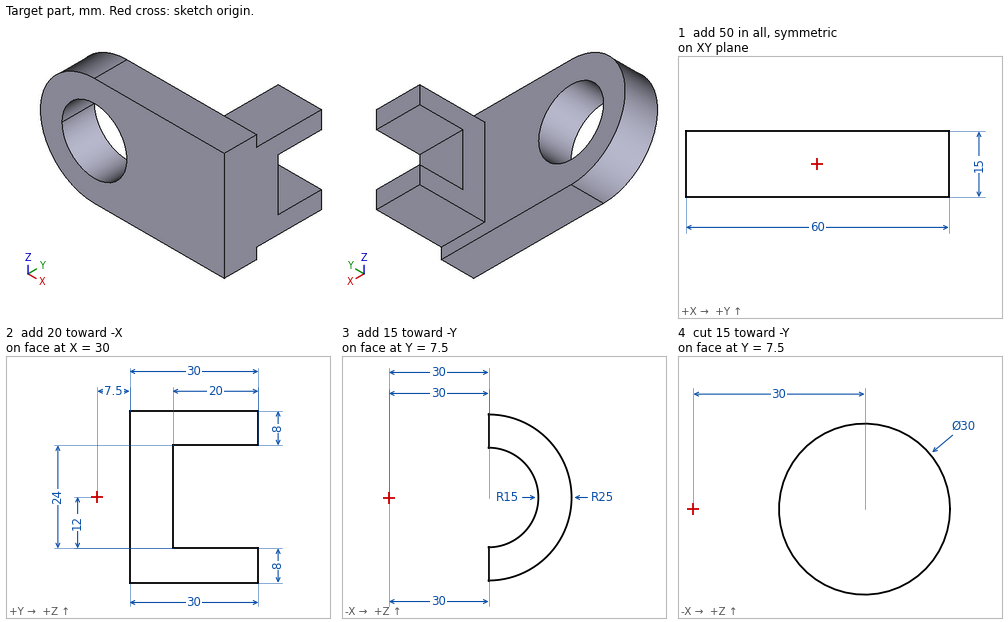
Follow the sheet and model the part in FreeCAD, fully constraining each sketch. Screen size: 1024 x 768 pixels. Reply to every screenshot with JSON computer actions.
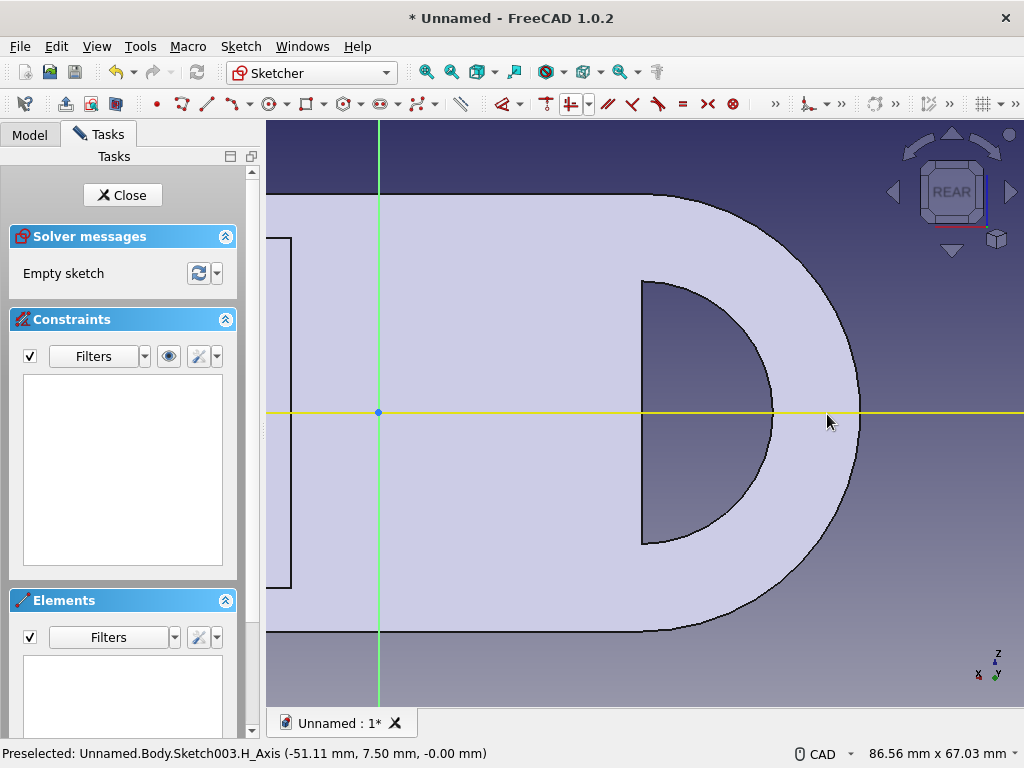
{"action": "key", "text": "g c"}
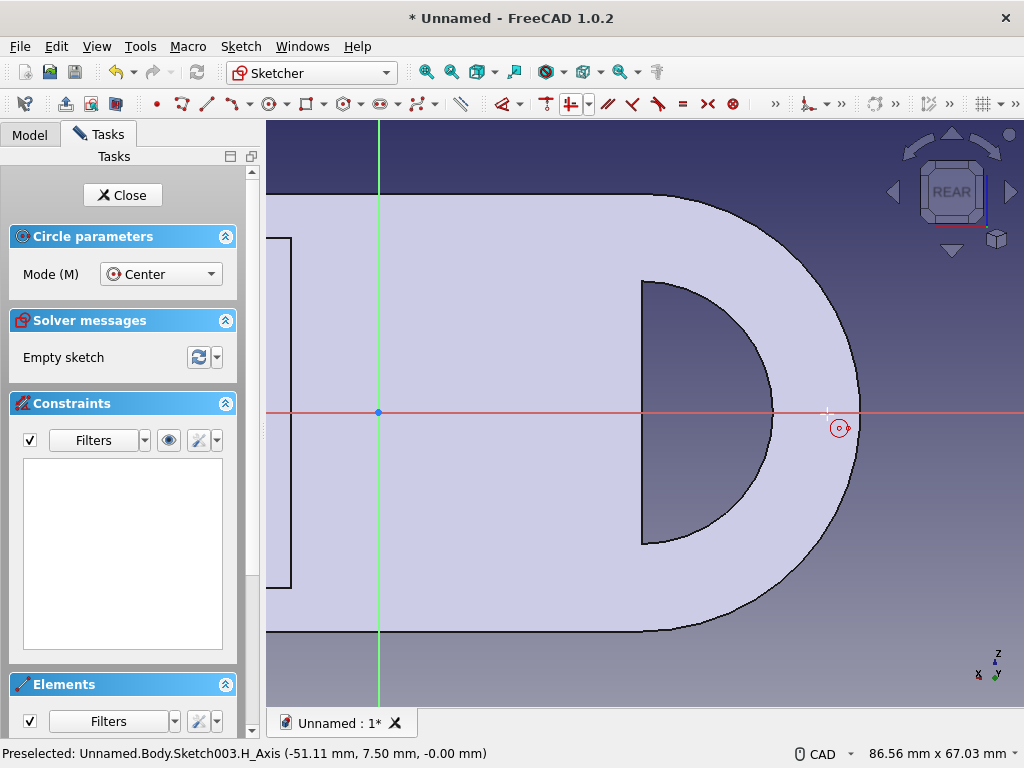
{"action": "left_click", "coordinate": [642, 413]}
{"action": "mouse_move", "coordinate": [734, 320]}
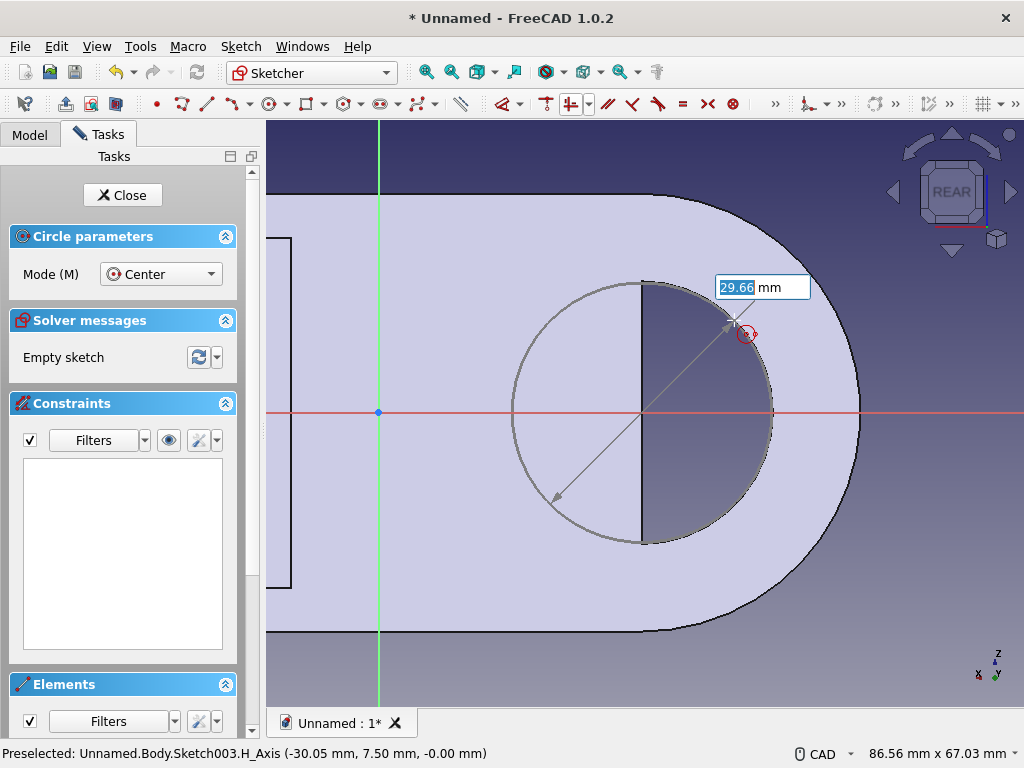
{"action": "type", "text": "30"}
{"action": "key", "text": "Return"}
{"action": "key", "text": "Escape"}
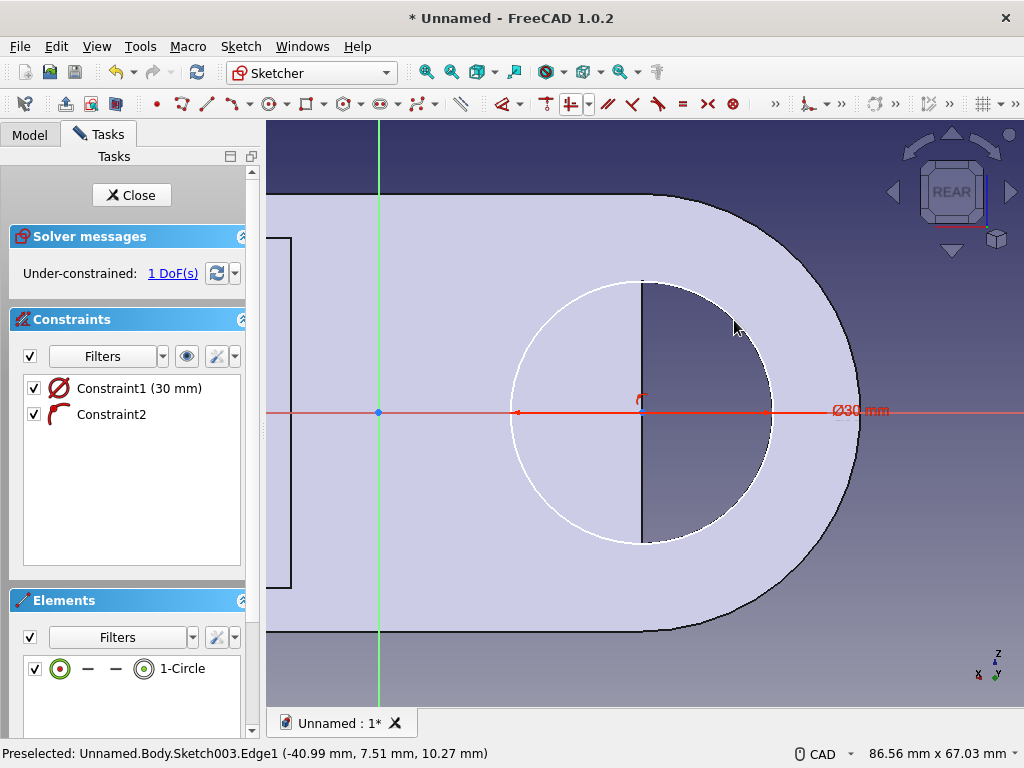
{"action": "key", "text": "d"}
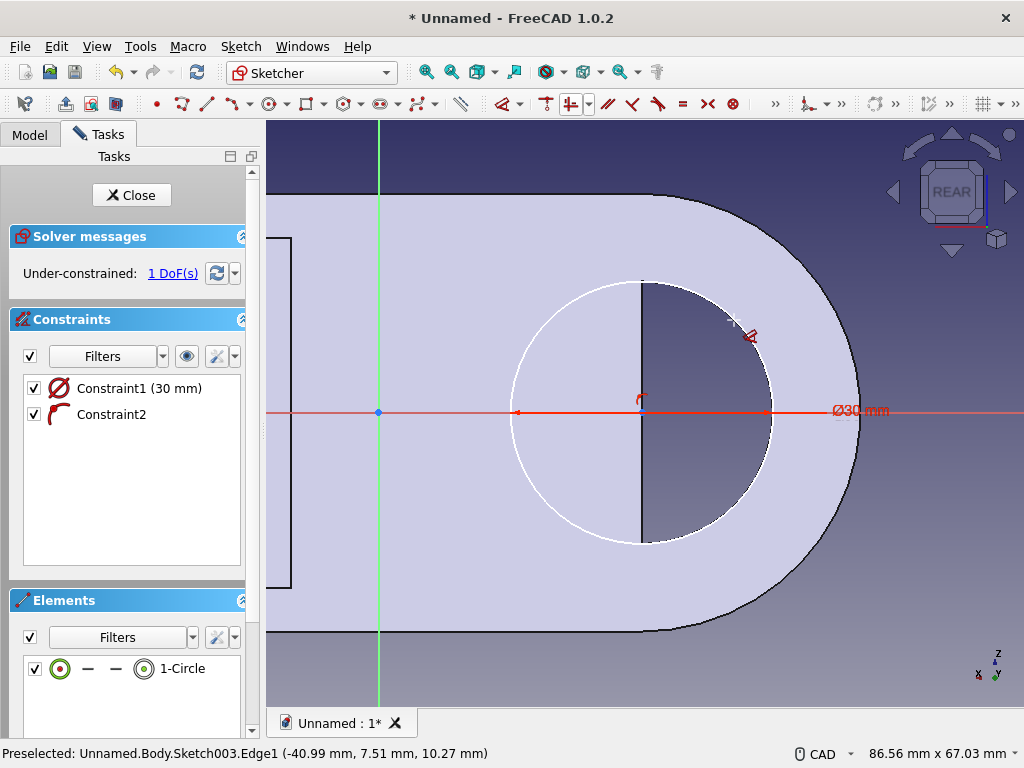
{"action": "left_click", "coordinate": [642, 413]}
{"action": "left_click", "coordinate": [450, 447]}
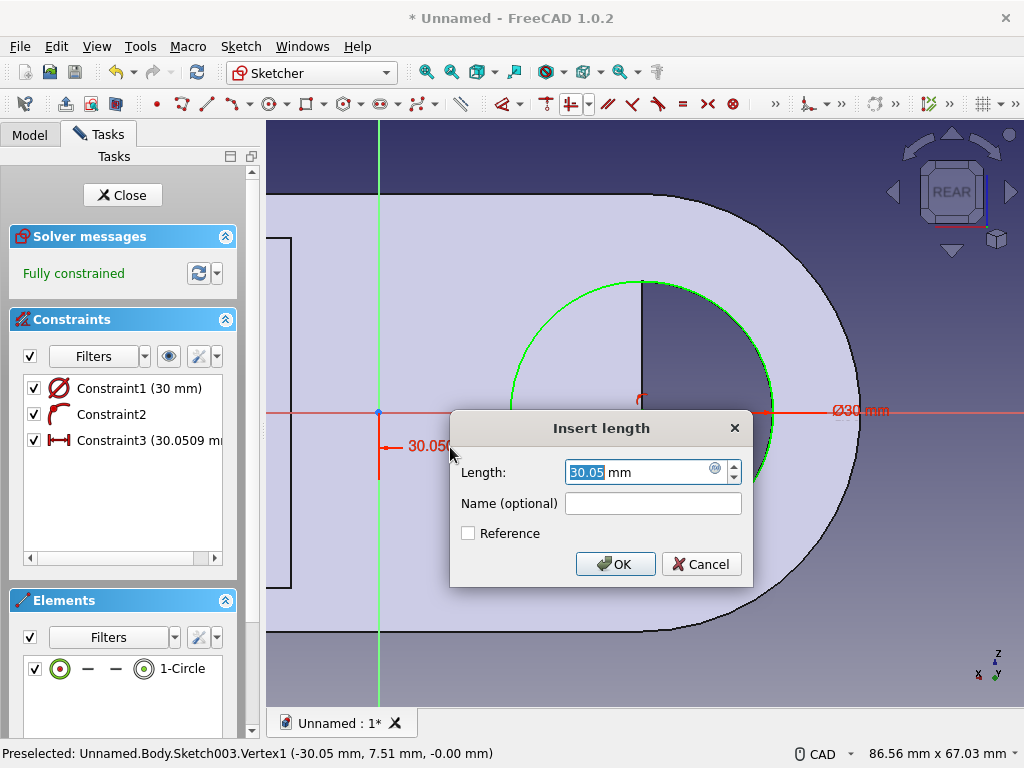
{"action": "type", "text": "30"}
{"action": "key", "text": "Return"}
{"action": "key", "text": "Escape"}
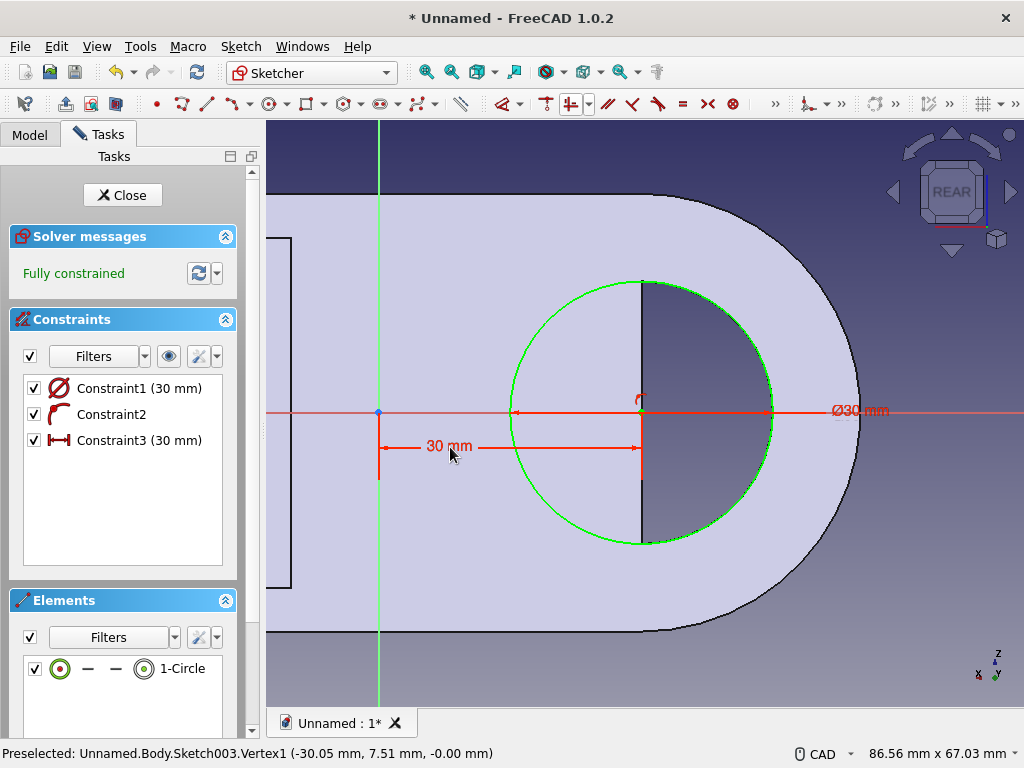
{"action": "left_click", "coordinate": [123, 195]}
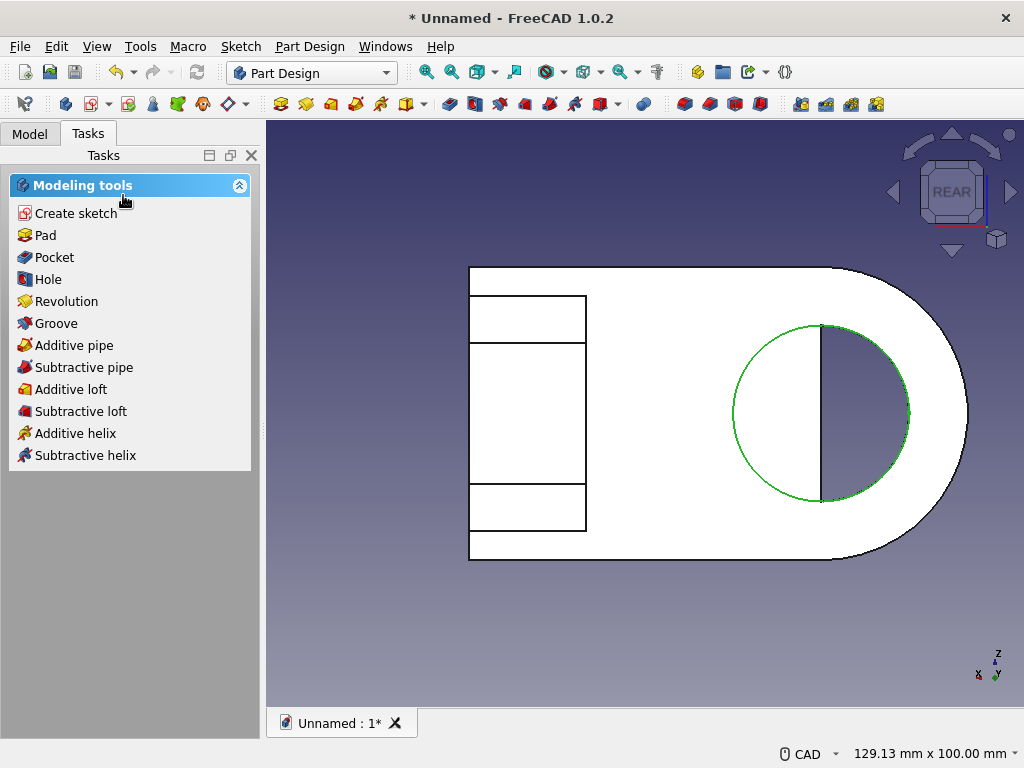
{"action": "left_click", "coordinate": [450, 104]}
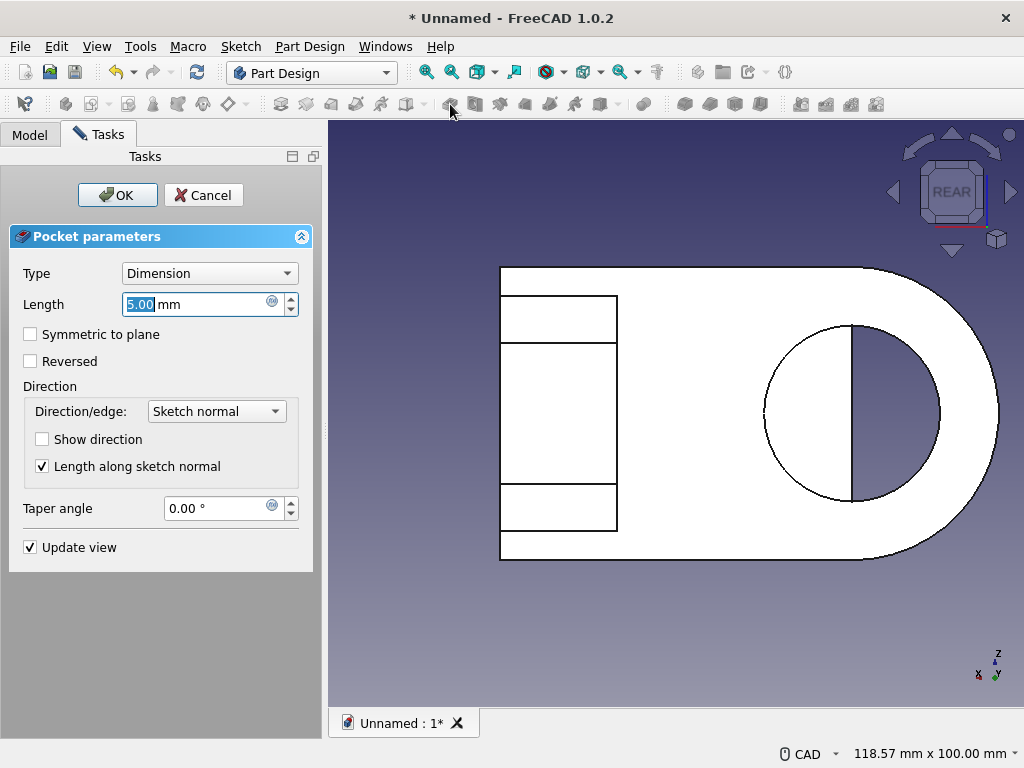
{"action": "type", "text": "15"}
{"action": "key", "text": "Tab"}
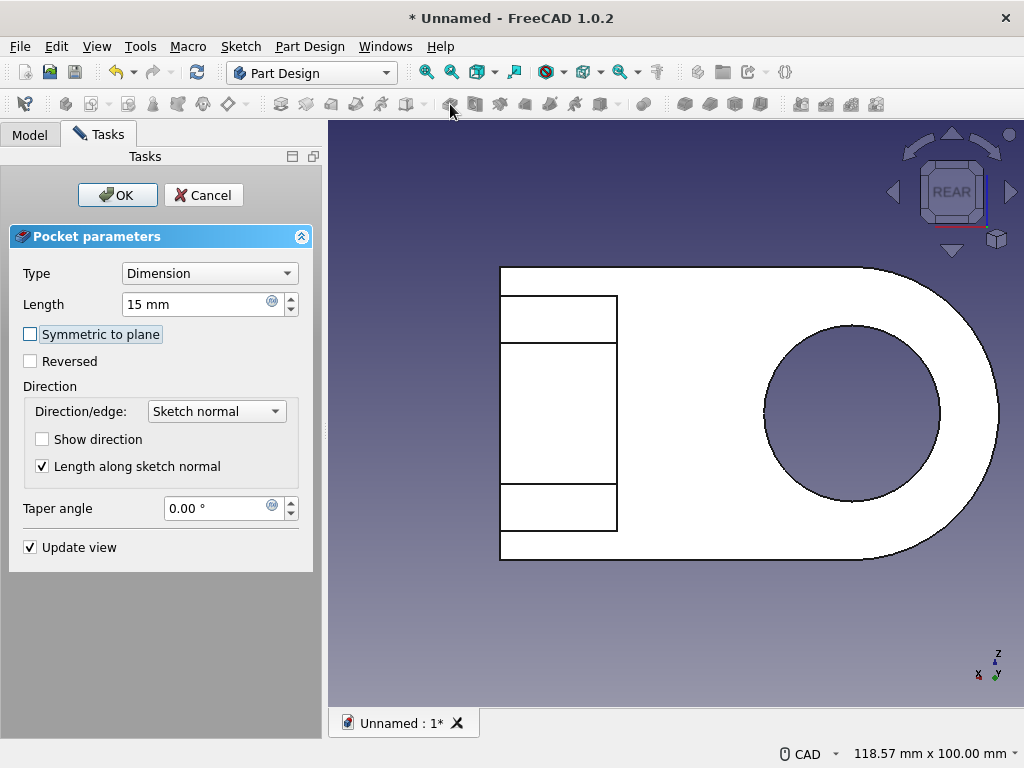
{"action": "left_click", "coordinate": [118, 195]}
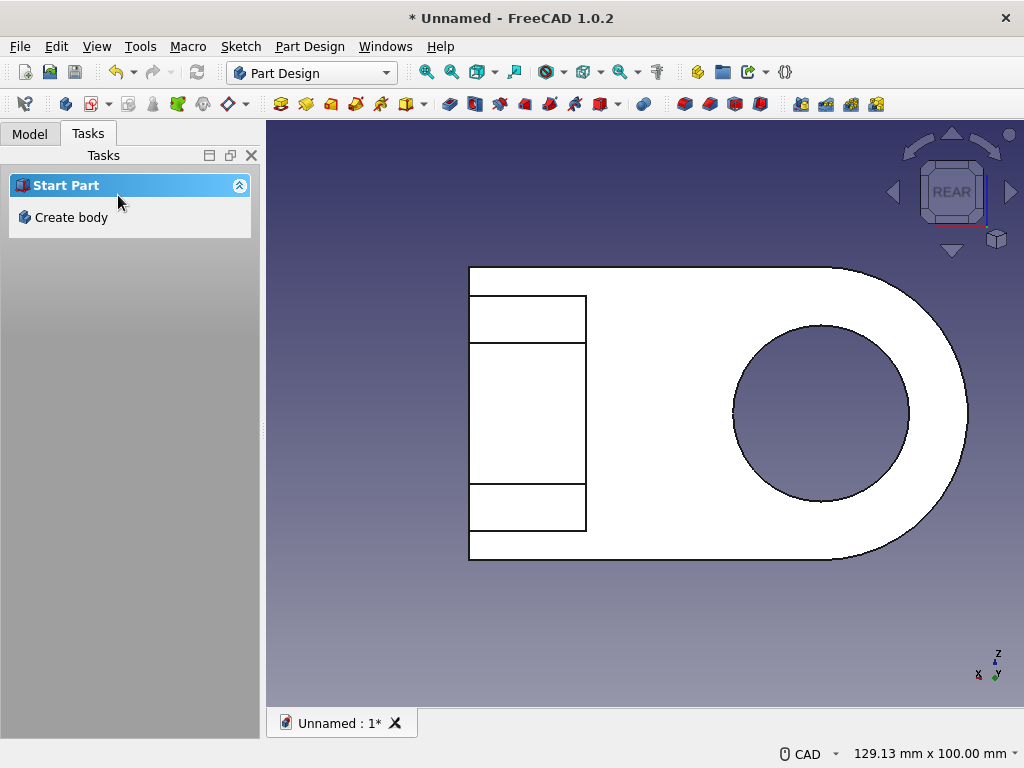
{"action": "key", "text": "0"}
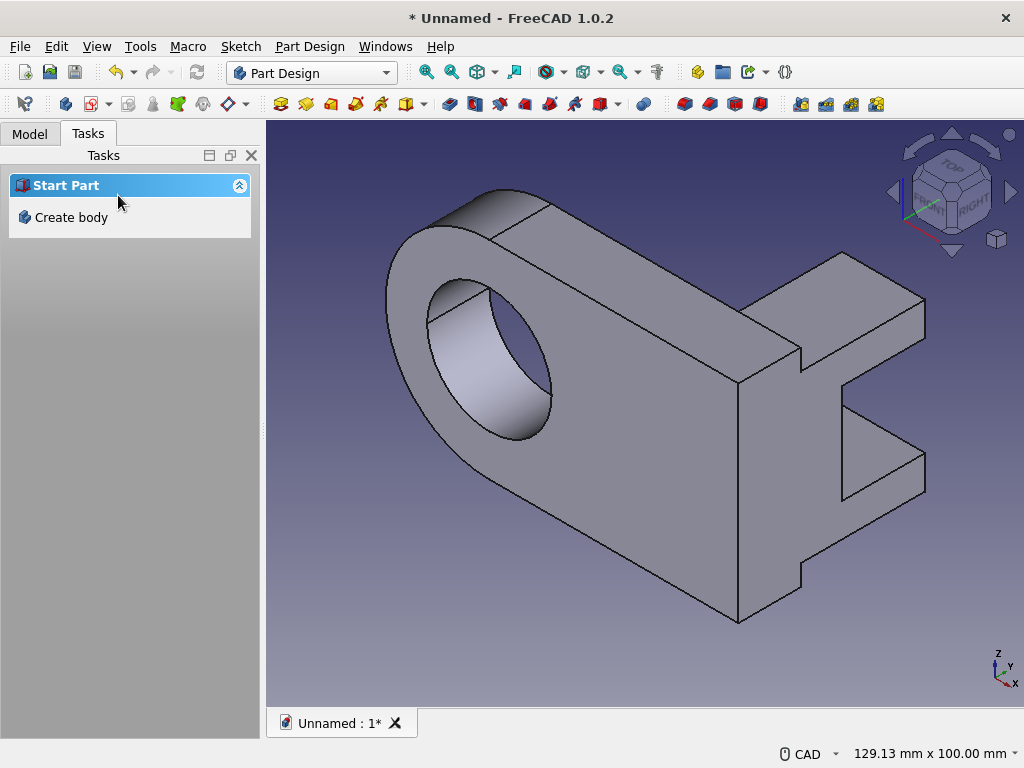
{"action": "left_click", "coordinate": [427, 72]}